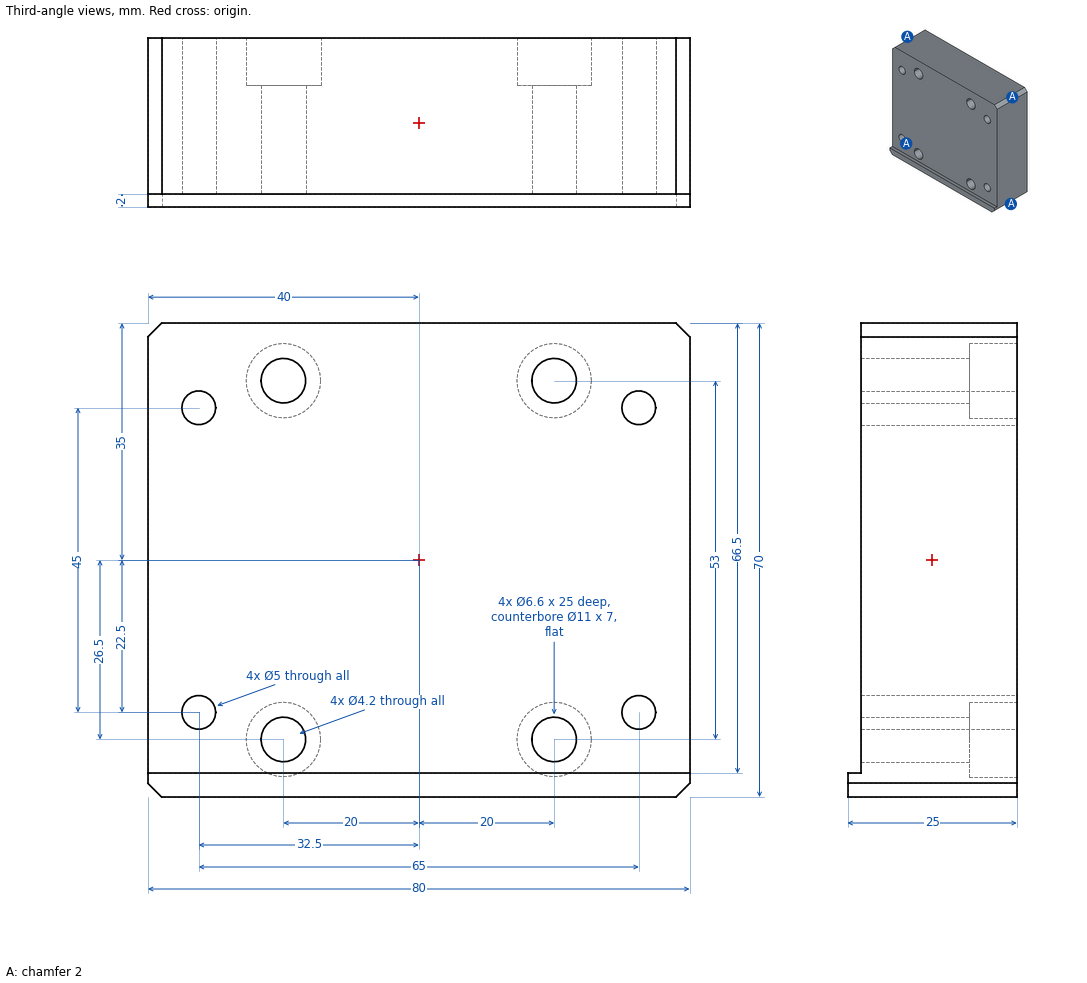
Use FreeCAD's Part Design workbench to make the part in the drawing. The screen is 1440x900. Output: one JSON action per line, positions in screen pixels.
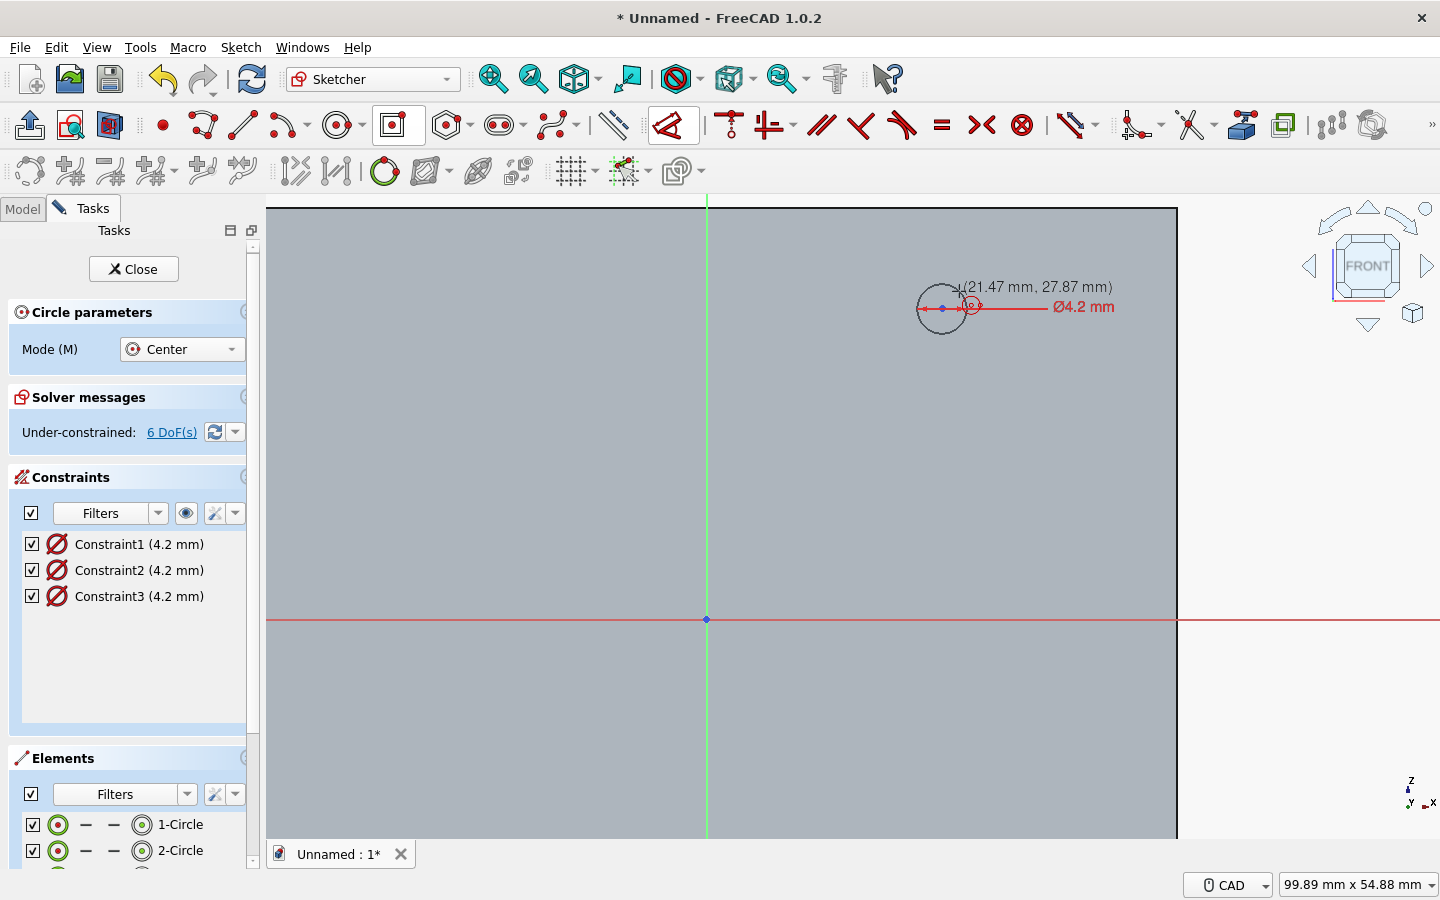
{"action": "left_click", "coordinate": [472, 308]}
{"action": "mouse_move", "coordinate": [489, 291]}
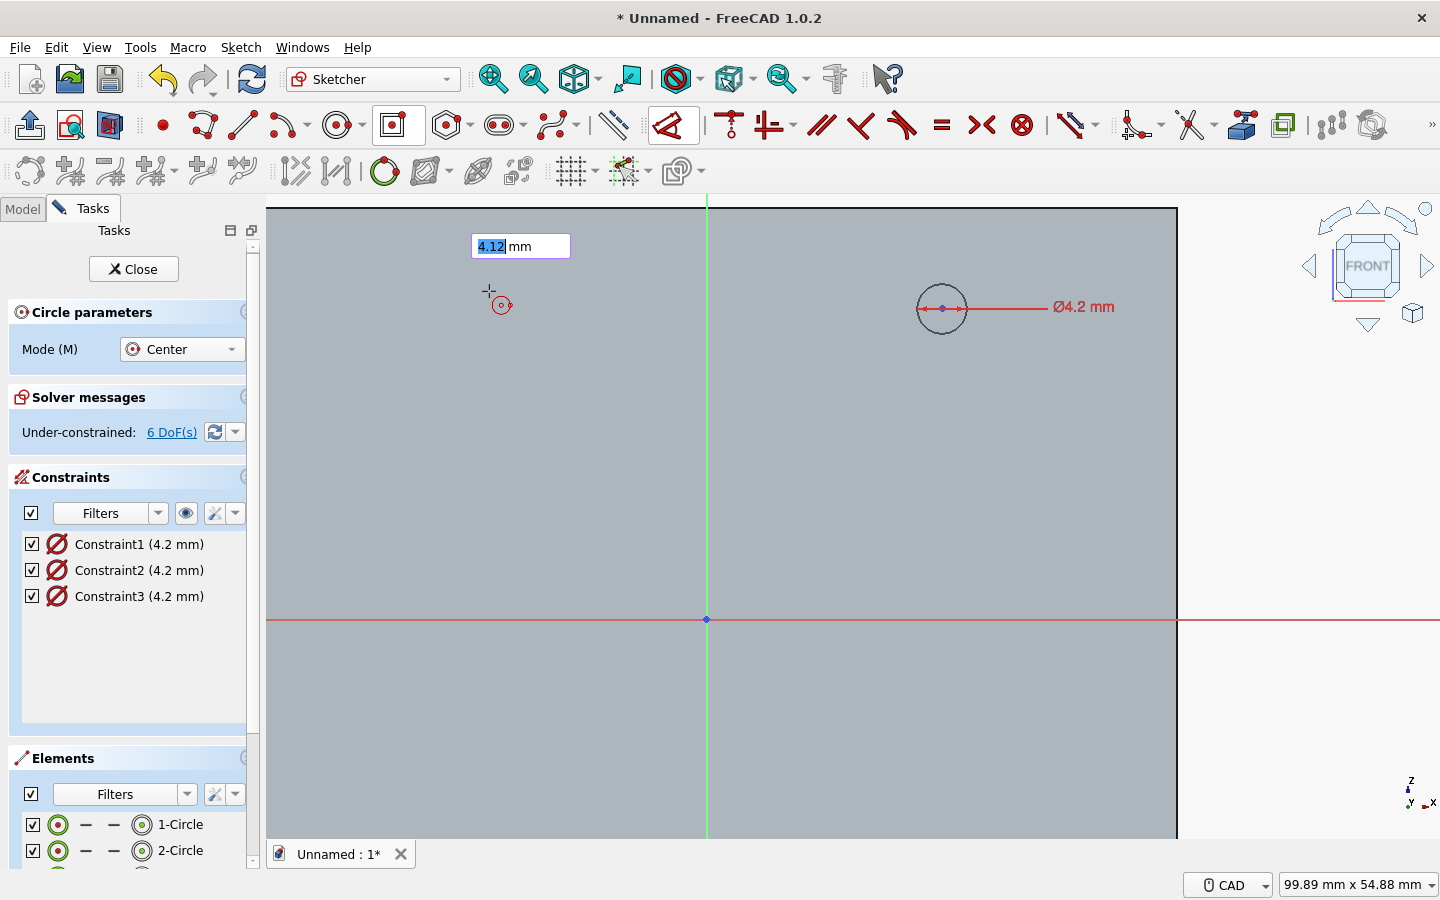
{"action": "type", "text": "4.2"}
{"action": "key", "text": "Return"}
{"action": "key", "text": "Escape"}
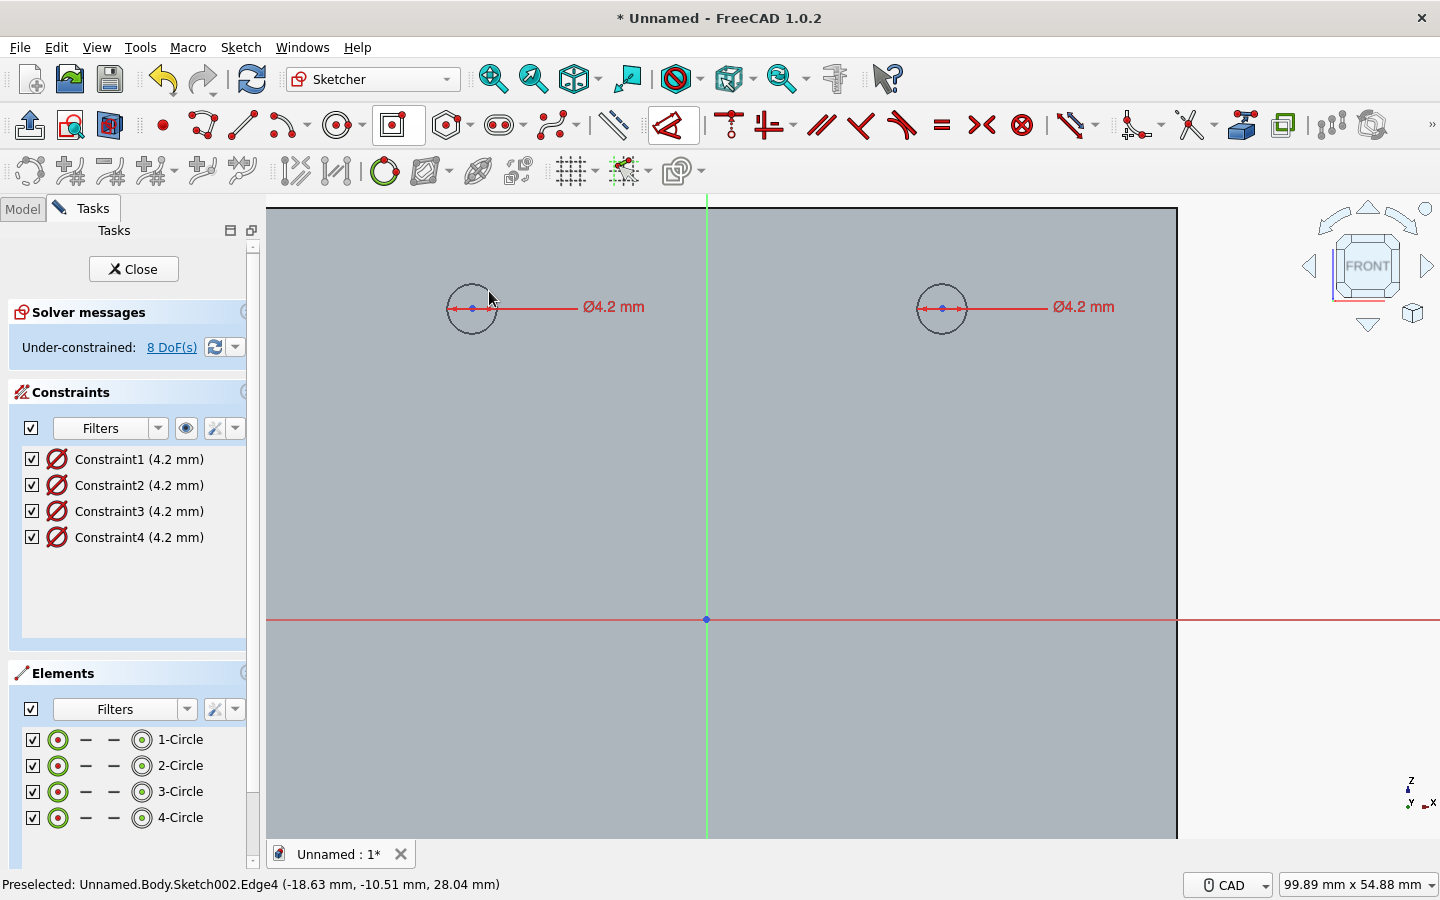
{"action": "scroll", "coordinate": [943, 307], "scroll_direction": "down", "scroll_amount": 2}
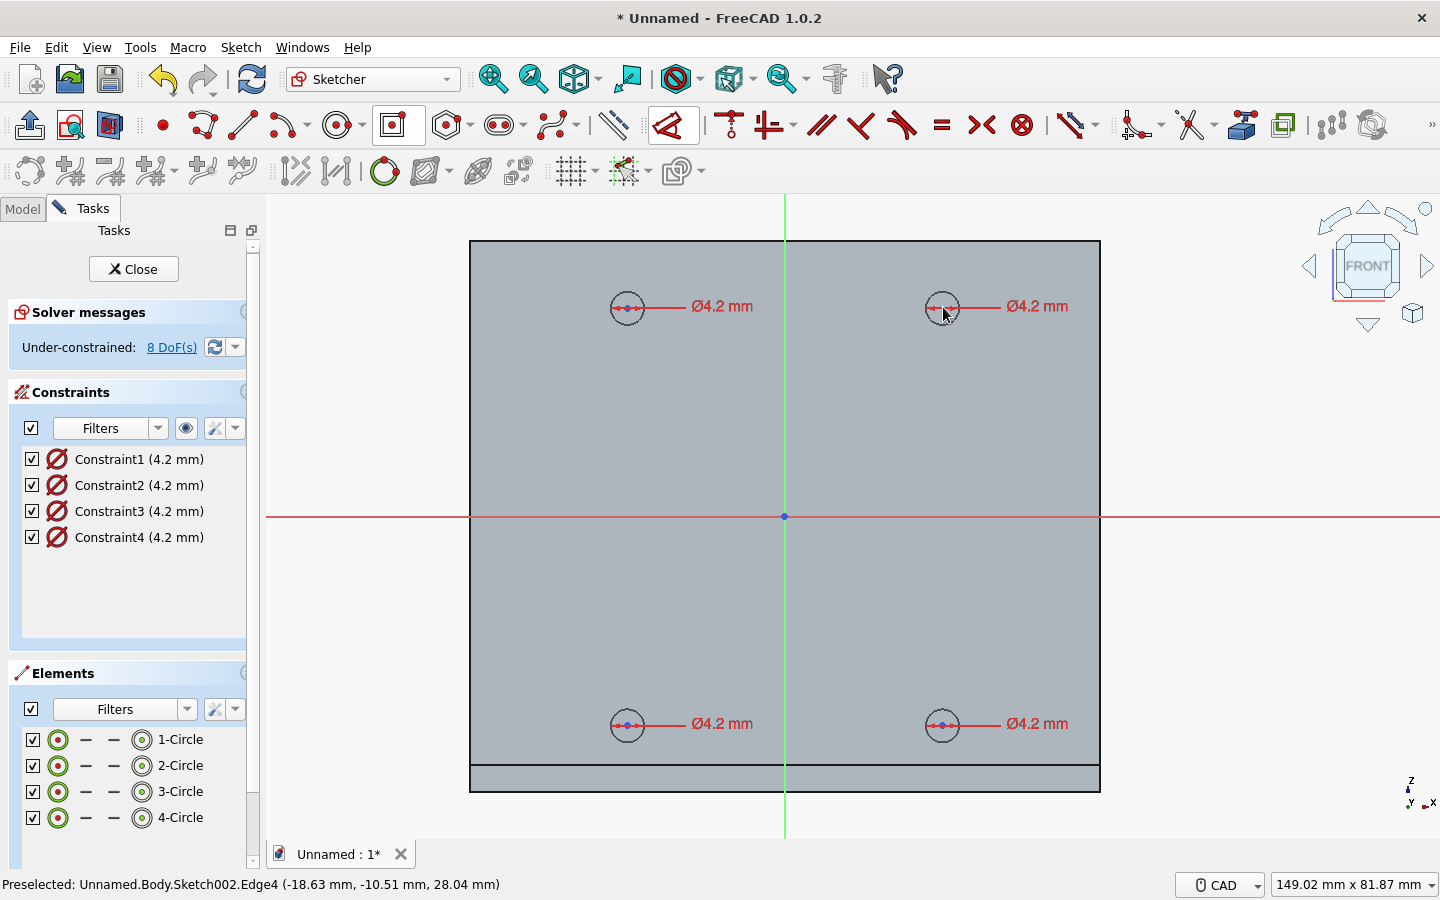
{"action": "left_click", "coordinate": [627, 726]}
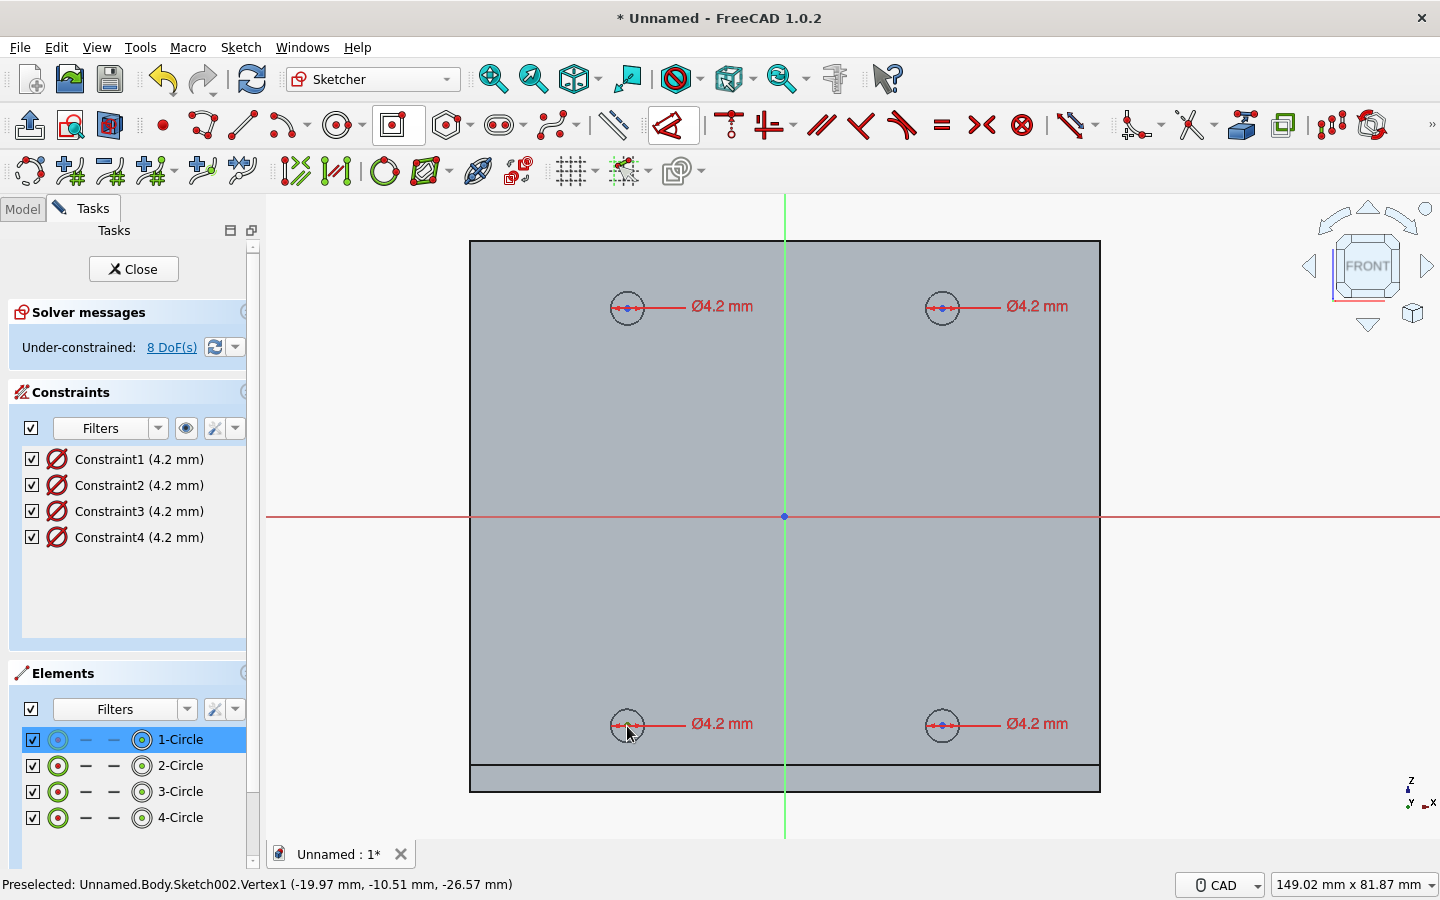
{"action": "left_click", "coordinate": [943, 726]}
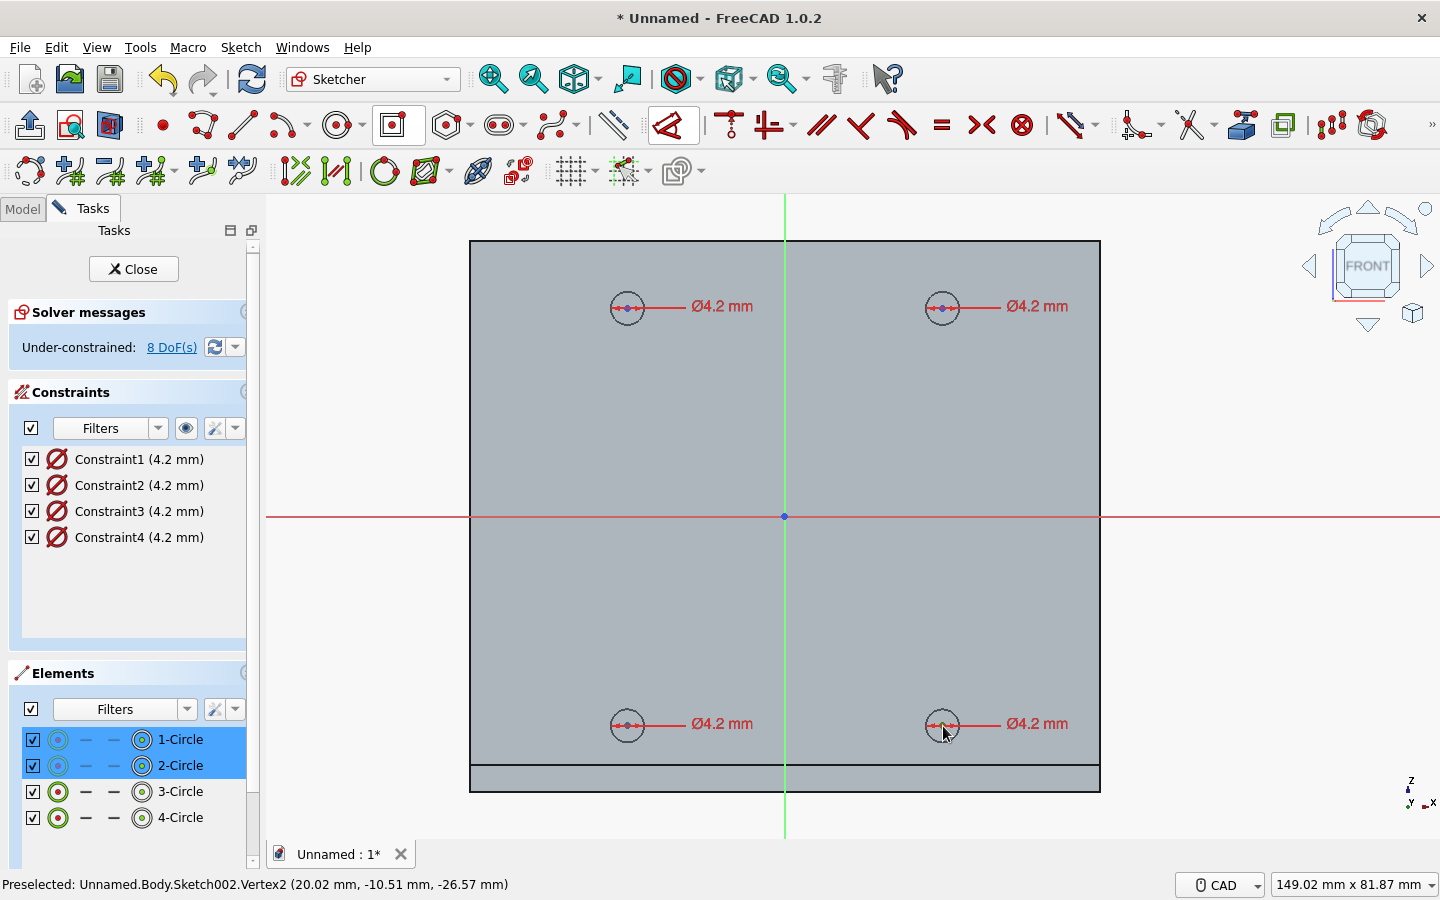
{"action": "left_click", "coordinate": [796, 126]}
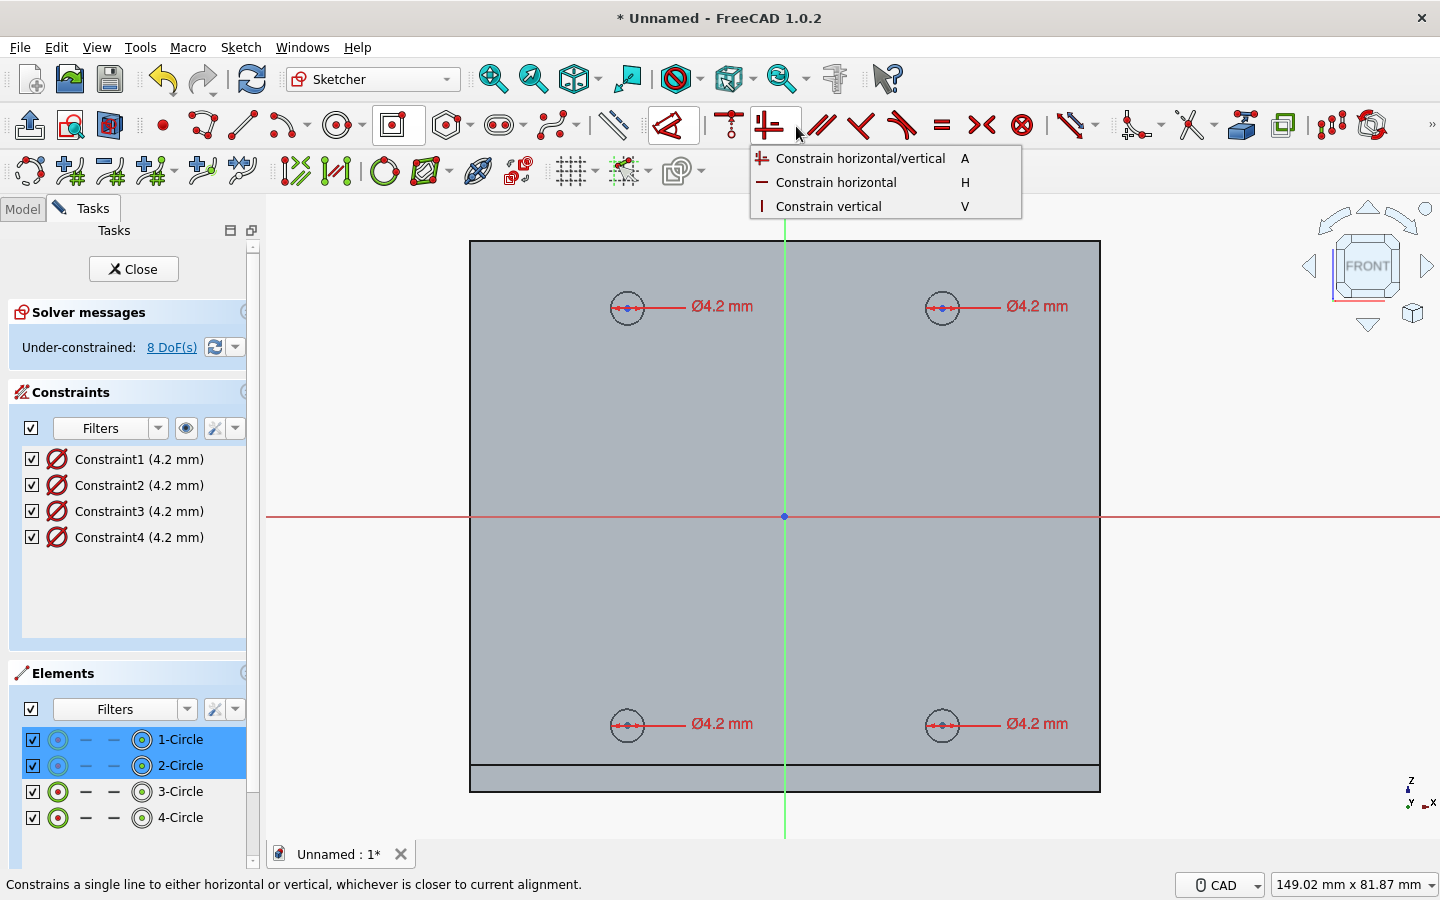
{"action": "left_click", "coordinate": [886, 182]}